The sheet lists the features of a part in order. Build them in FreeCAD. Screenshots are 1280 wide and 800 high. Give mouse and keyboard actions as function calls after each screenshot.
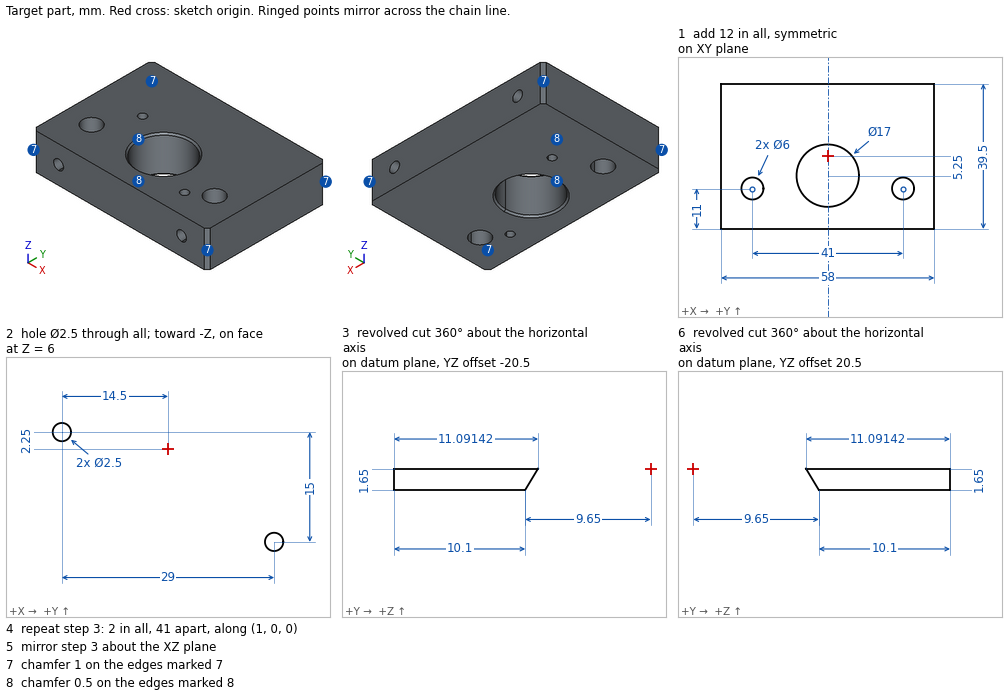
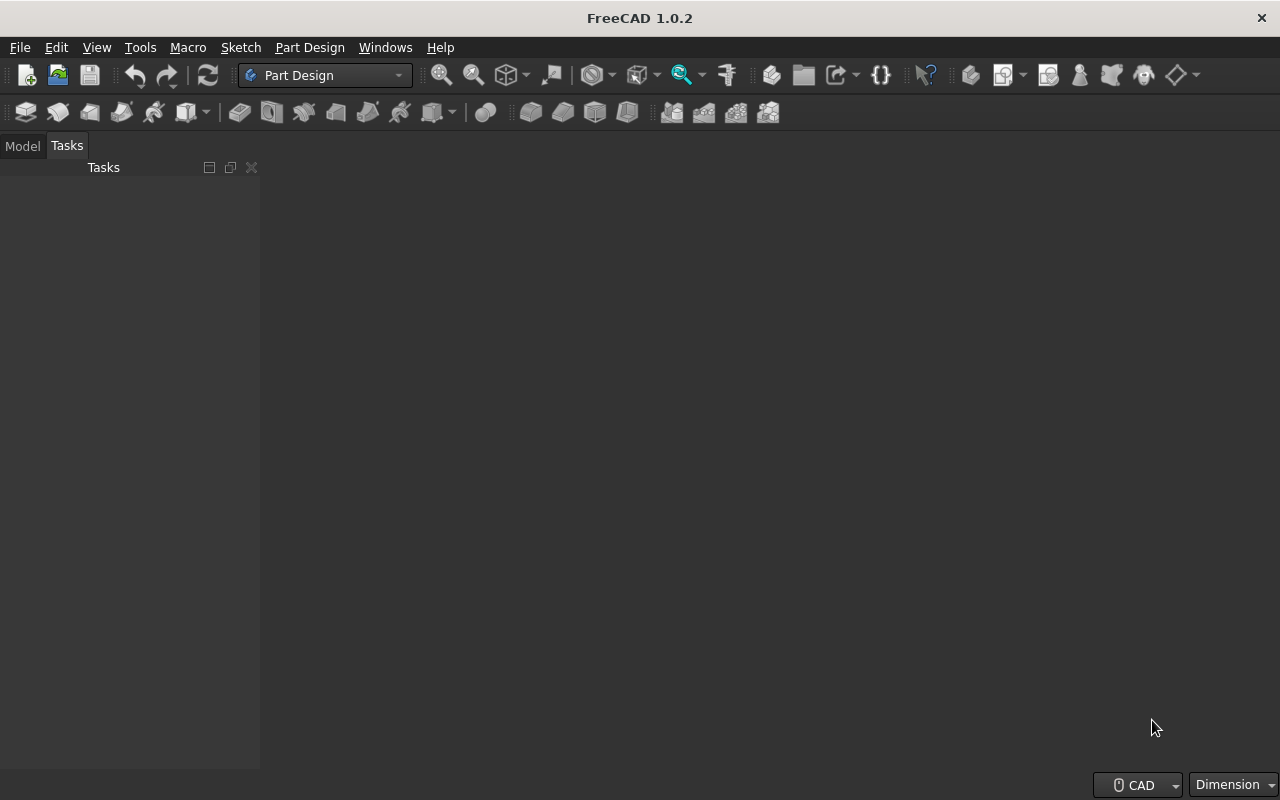
key(ctrl+n)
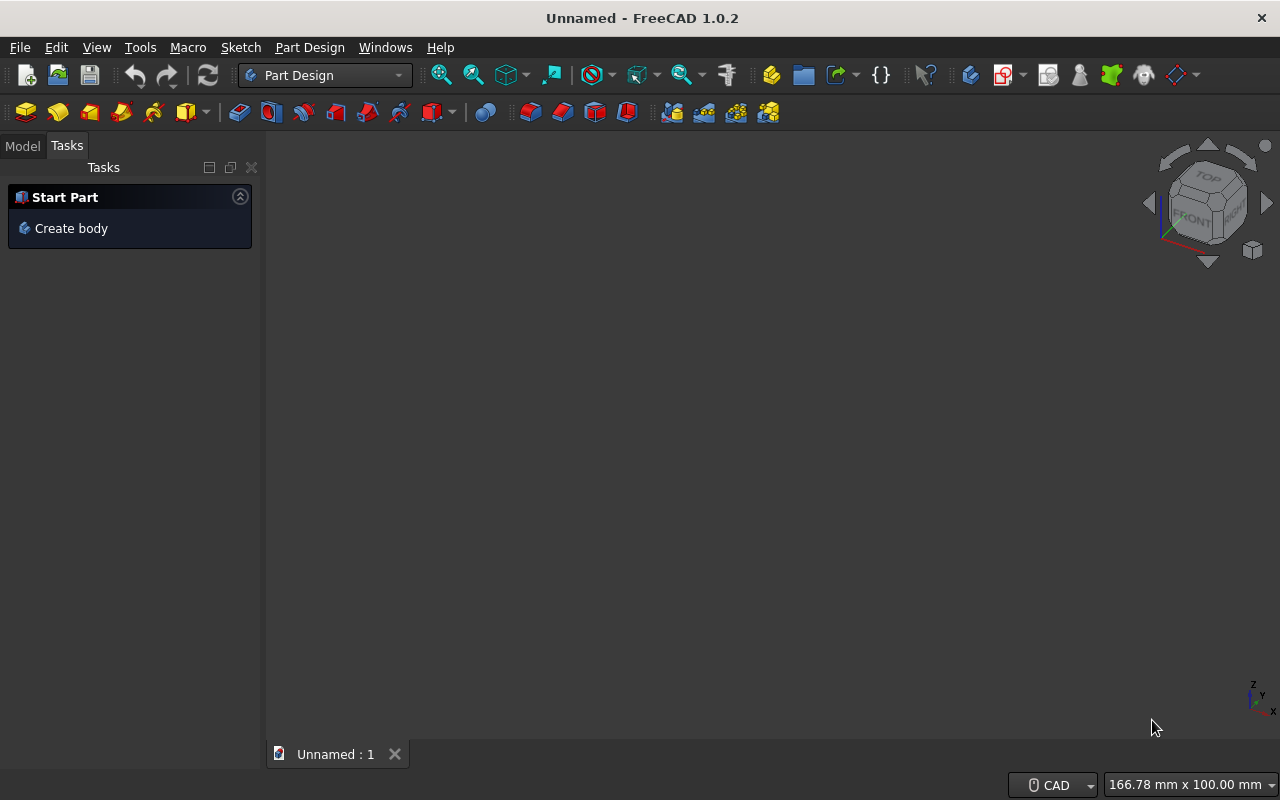
click(1004, 76)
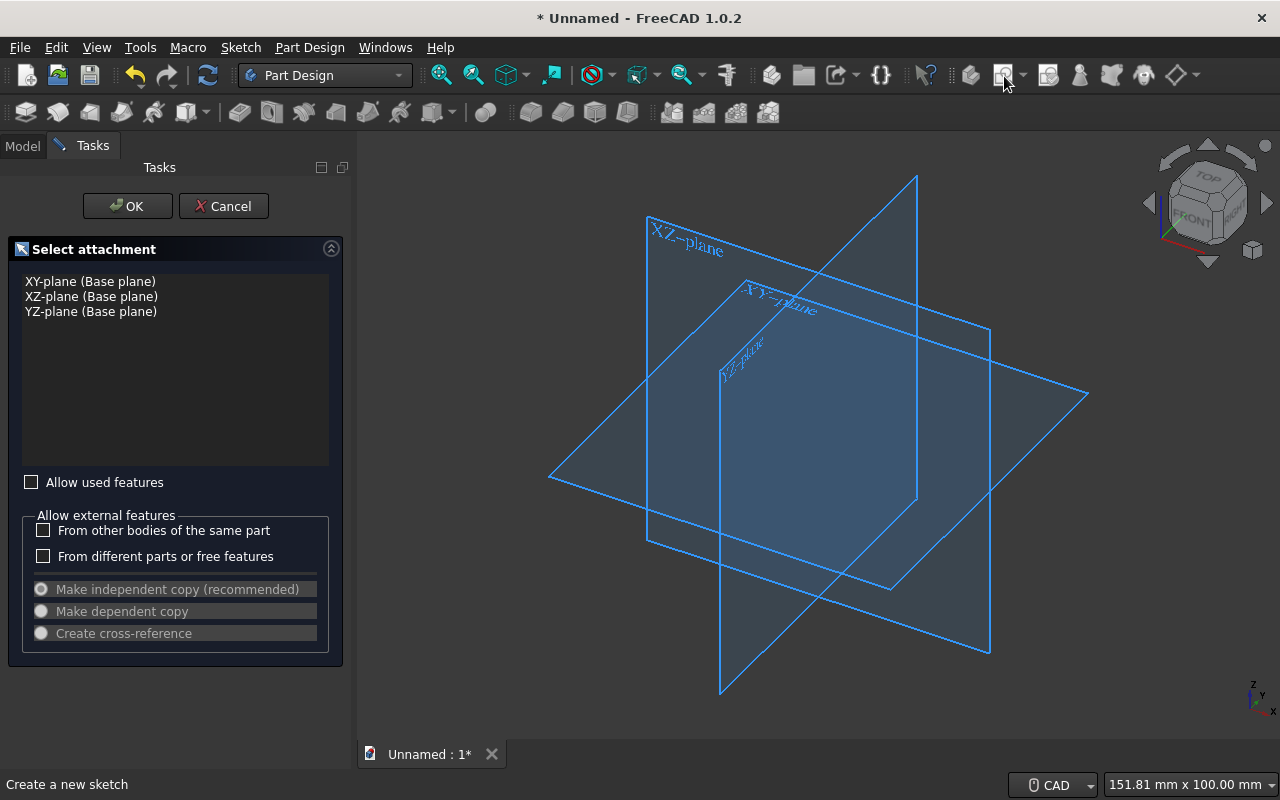
click(82, 282)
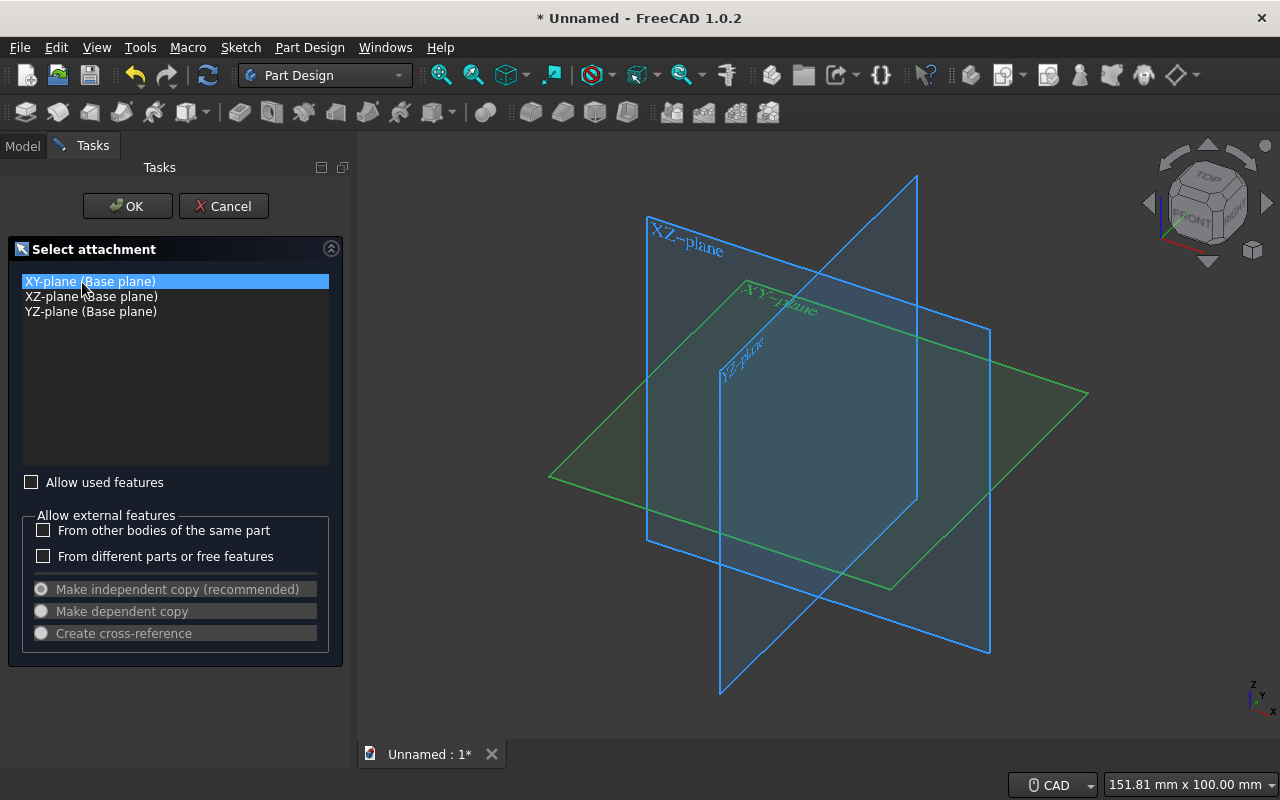
click(128, 206)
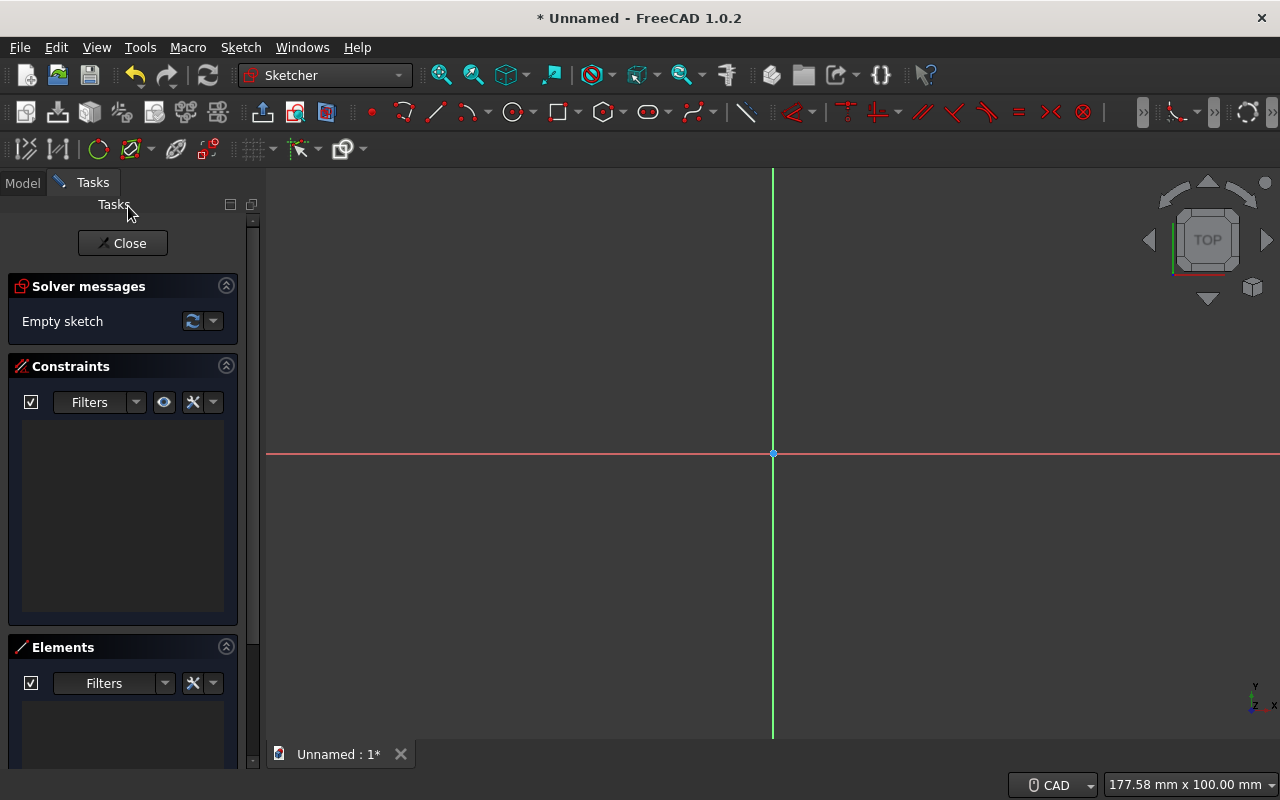
scroll(912, 454, up, 2)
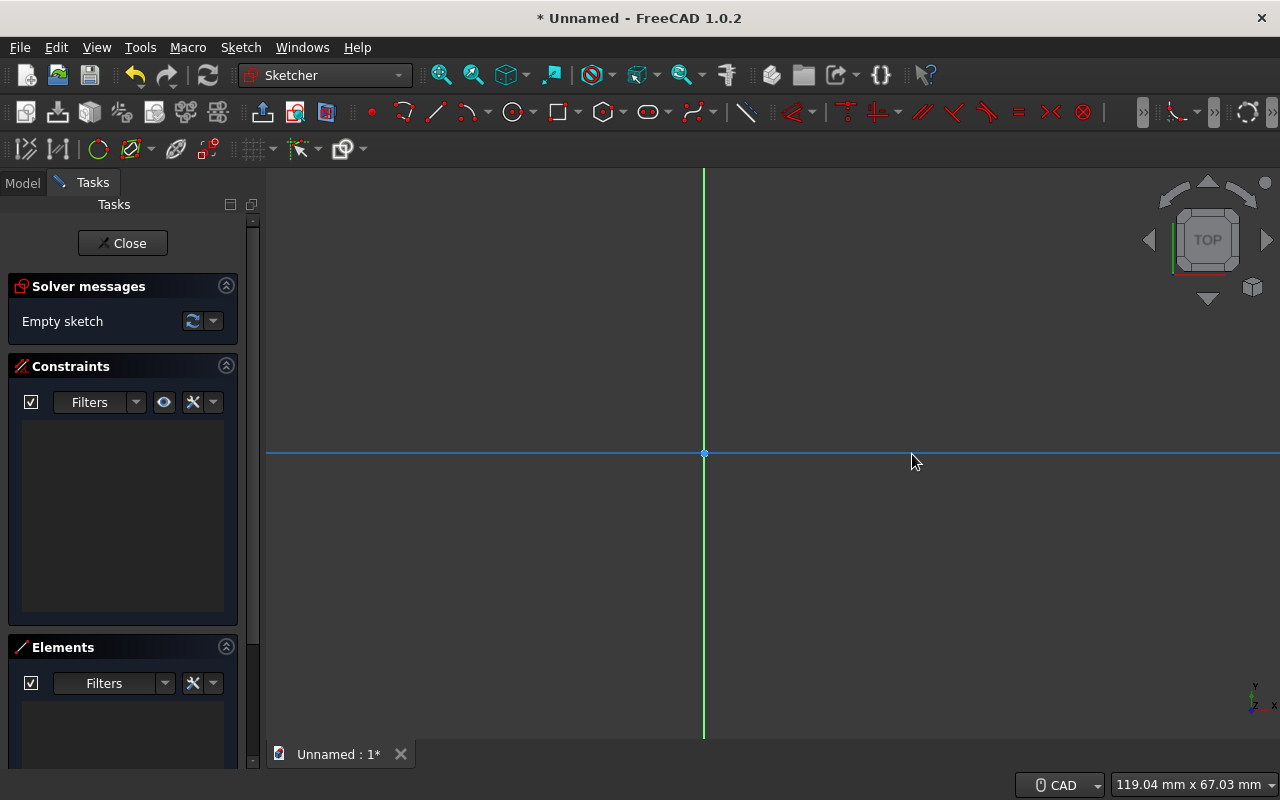
key(g)
key(v)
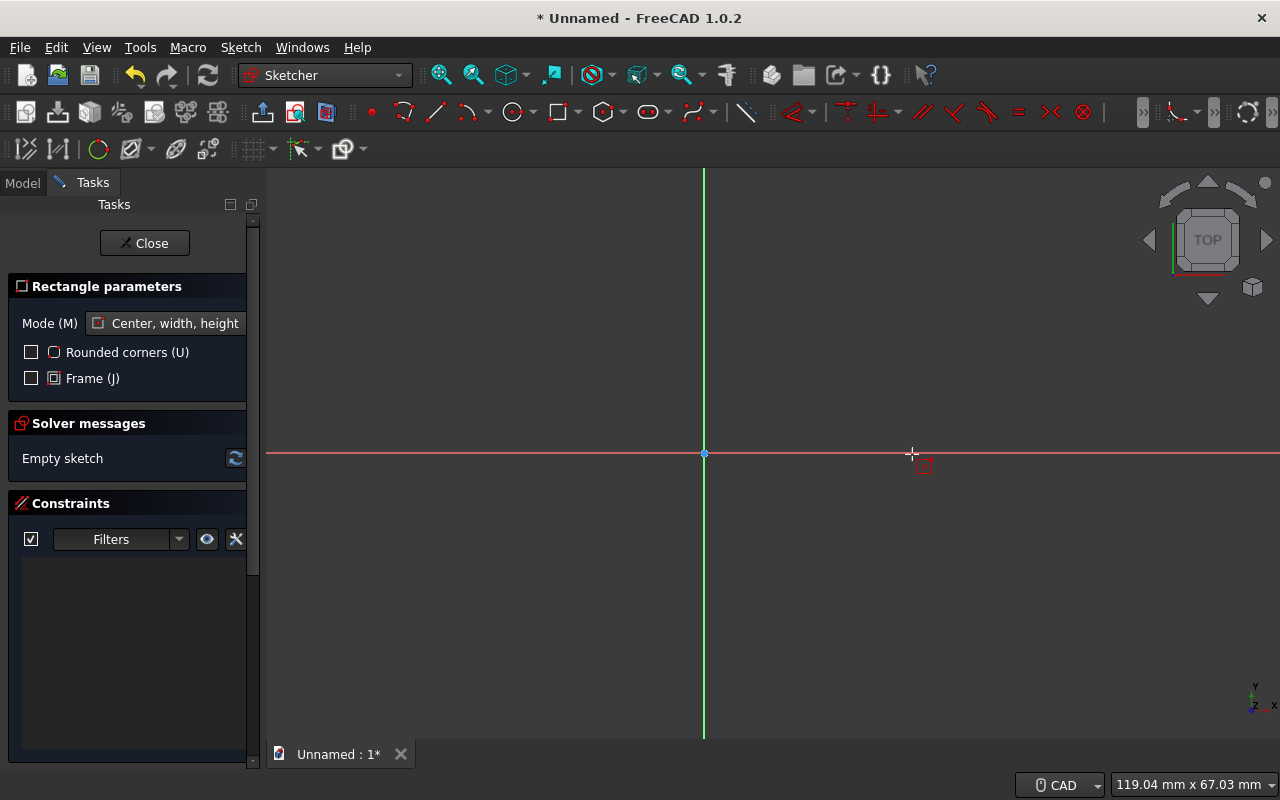
click(704, 453)
click(951, 285)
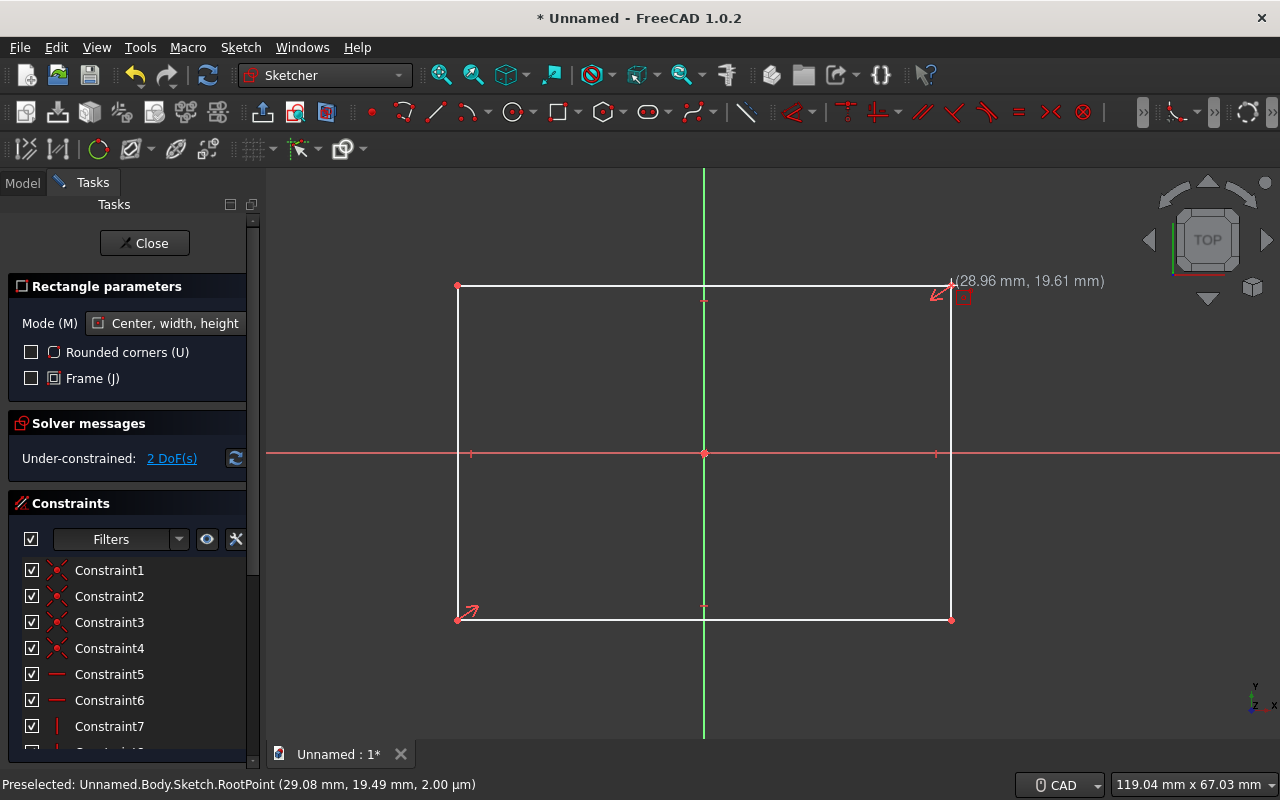
key(g)
key(c)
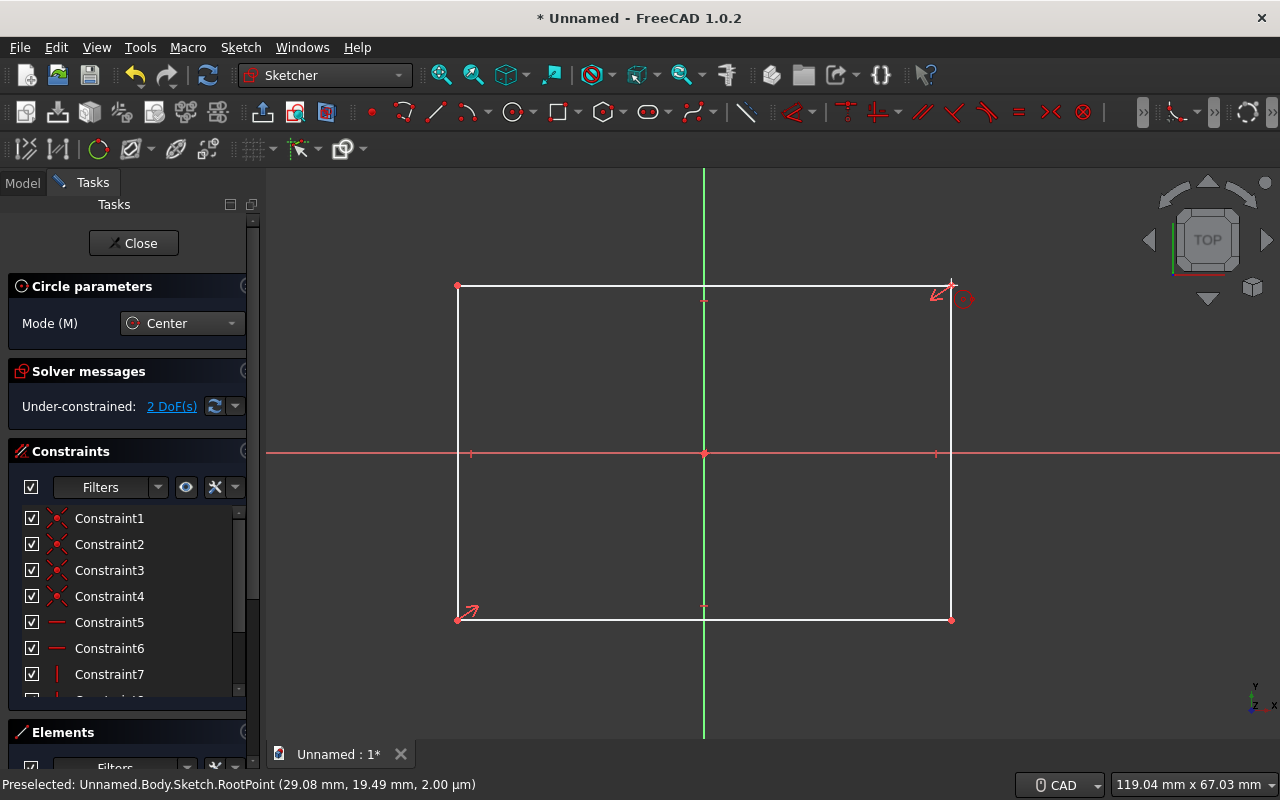
click(530, 528)
click(548, 509)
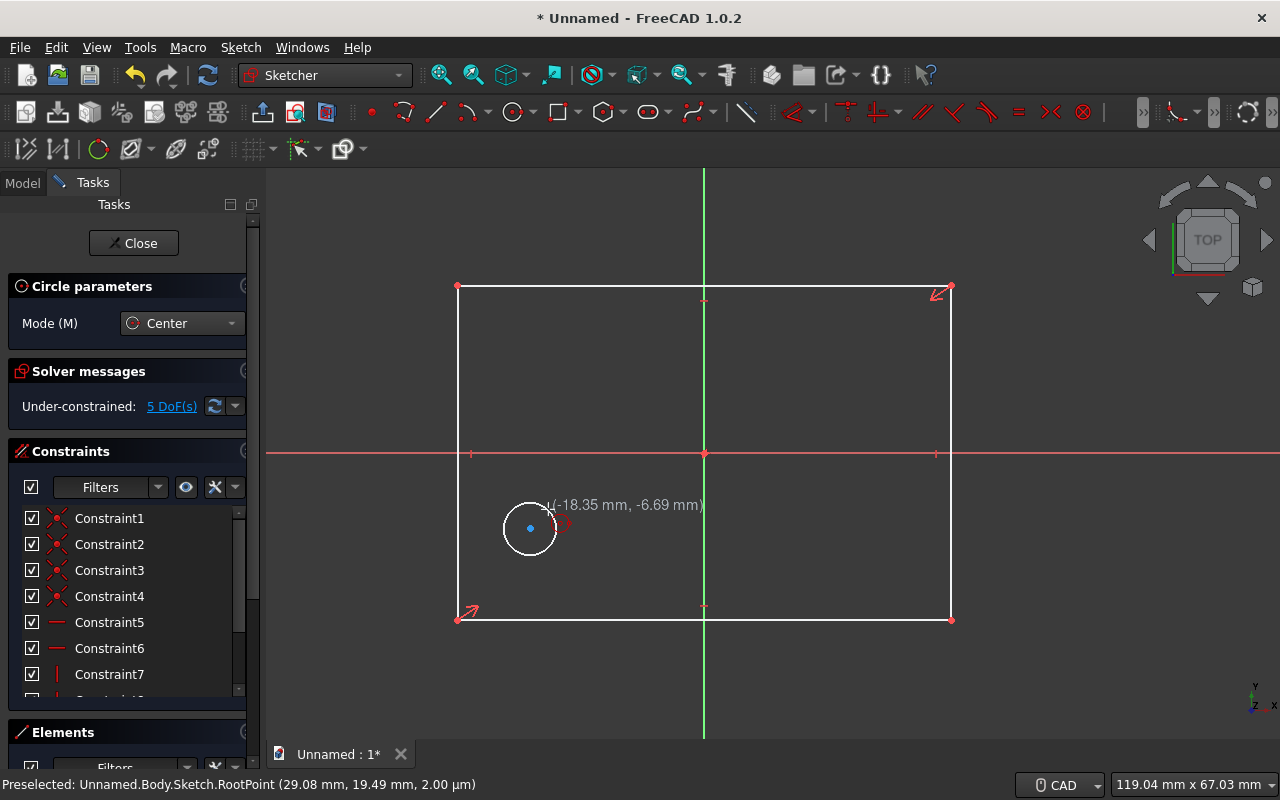
click(879, 528)
click(897, 509)